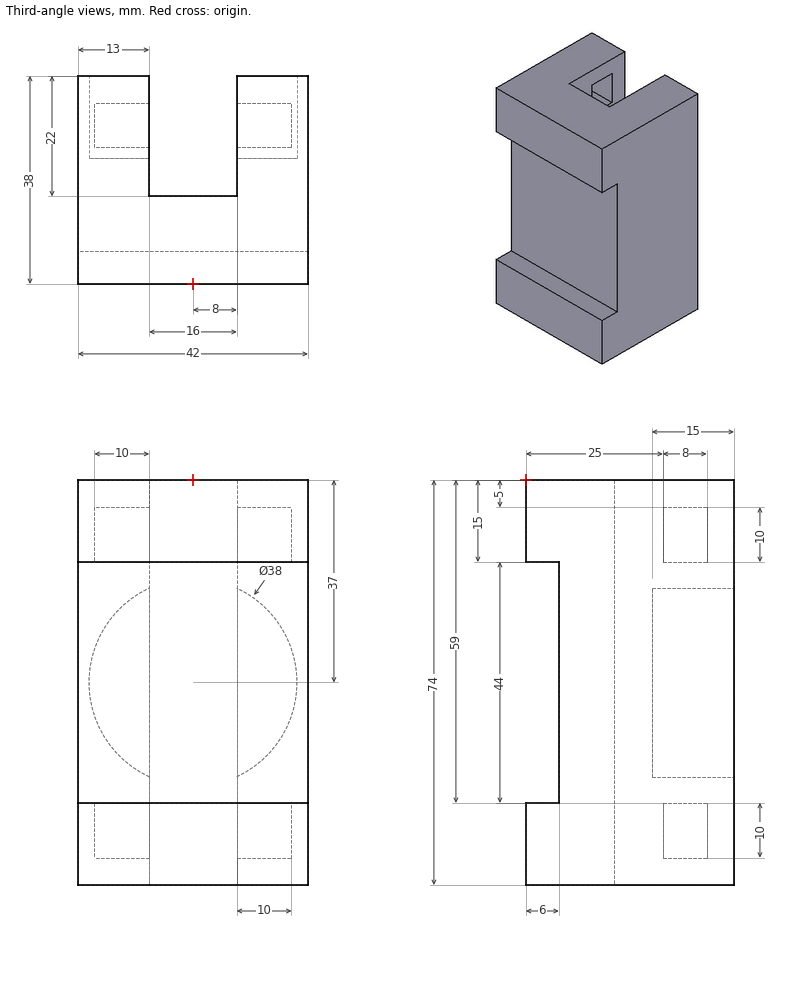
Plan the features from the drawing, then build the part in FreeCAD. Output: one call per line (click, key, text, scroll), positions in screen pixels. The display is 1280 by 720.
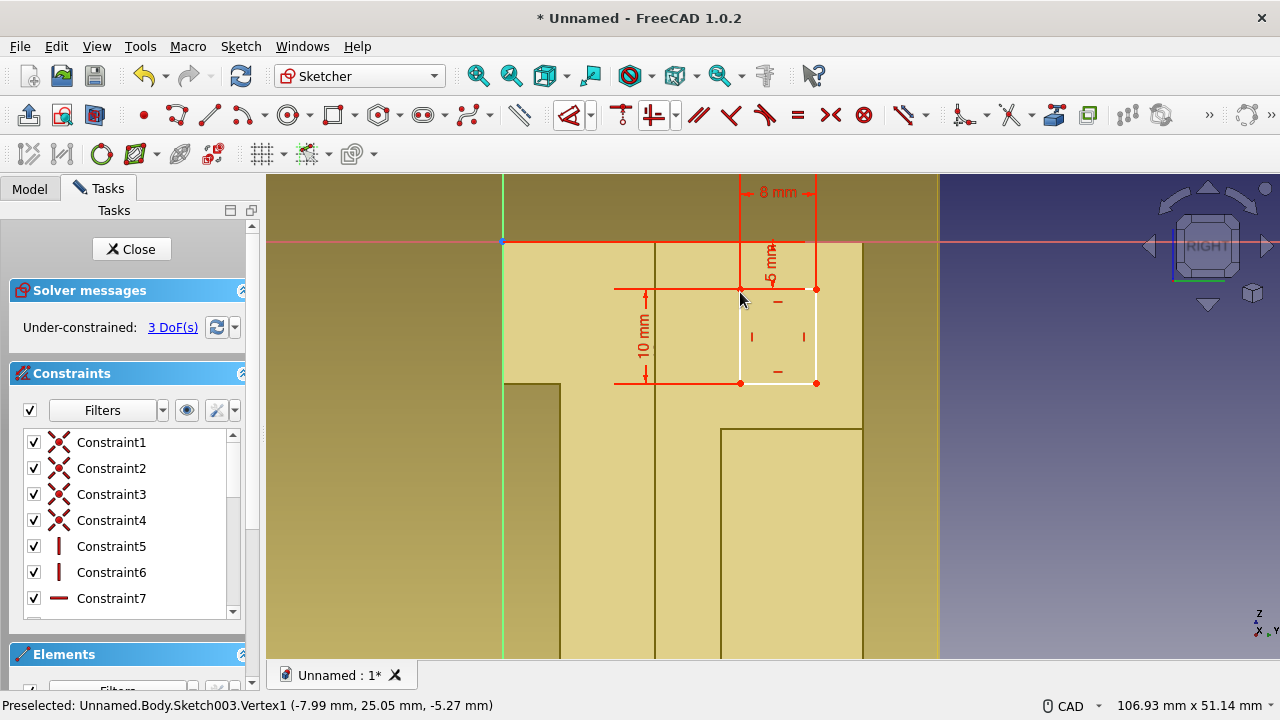
click(740, 289)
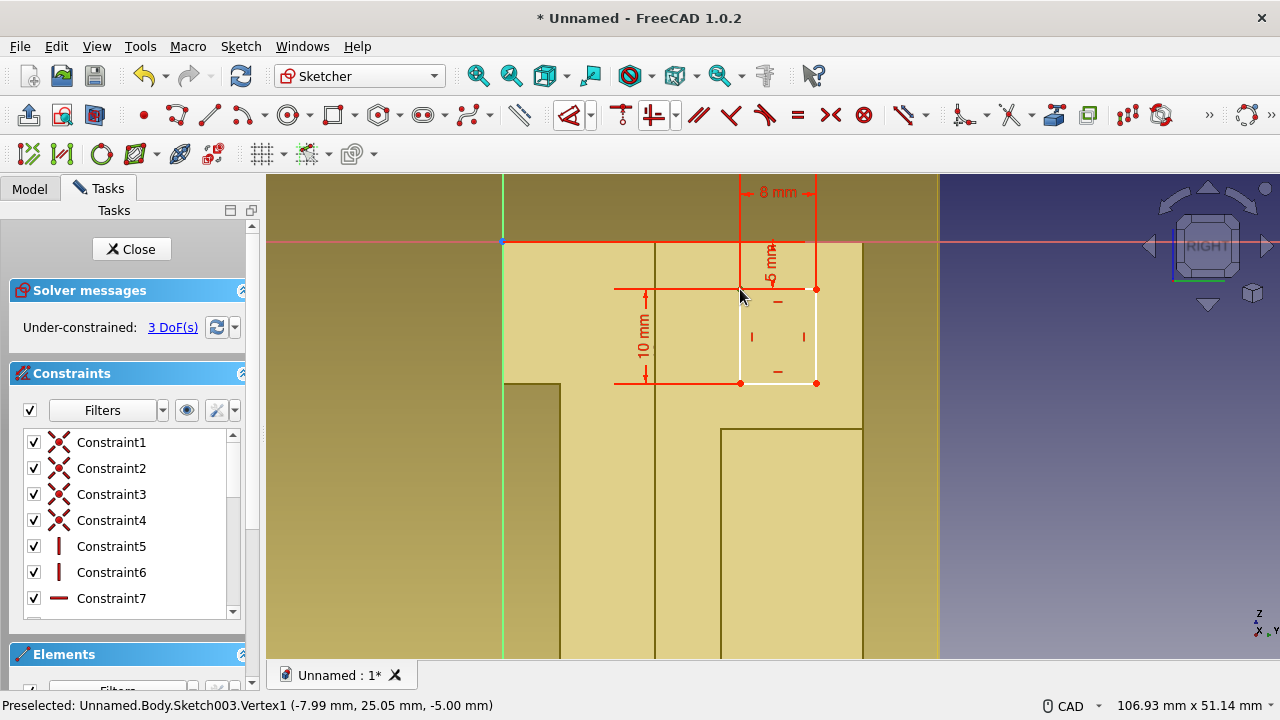
key(l)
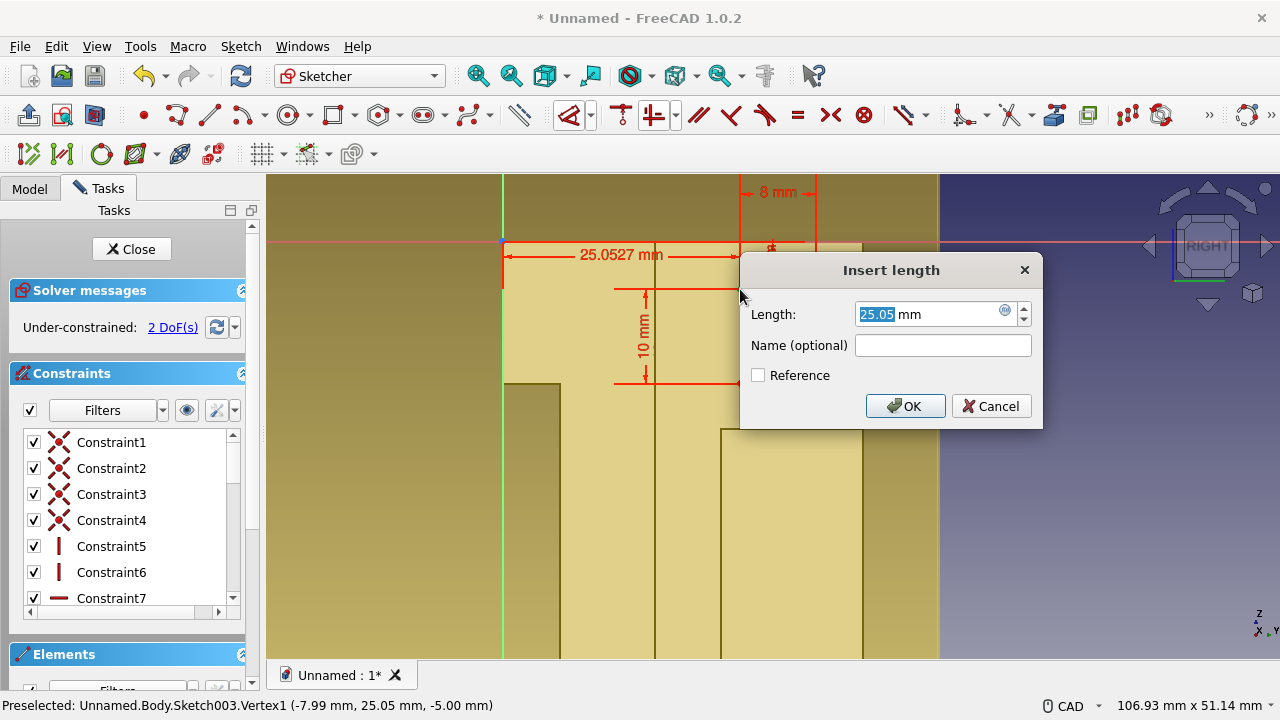
text(25)
key(Return)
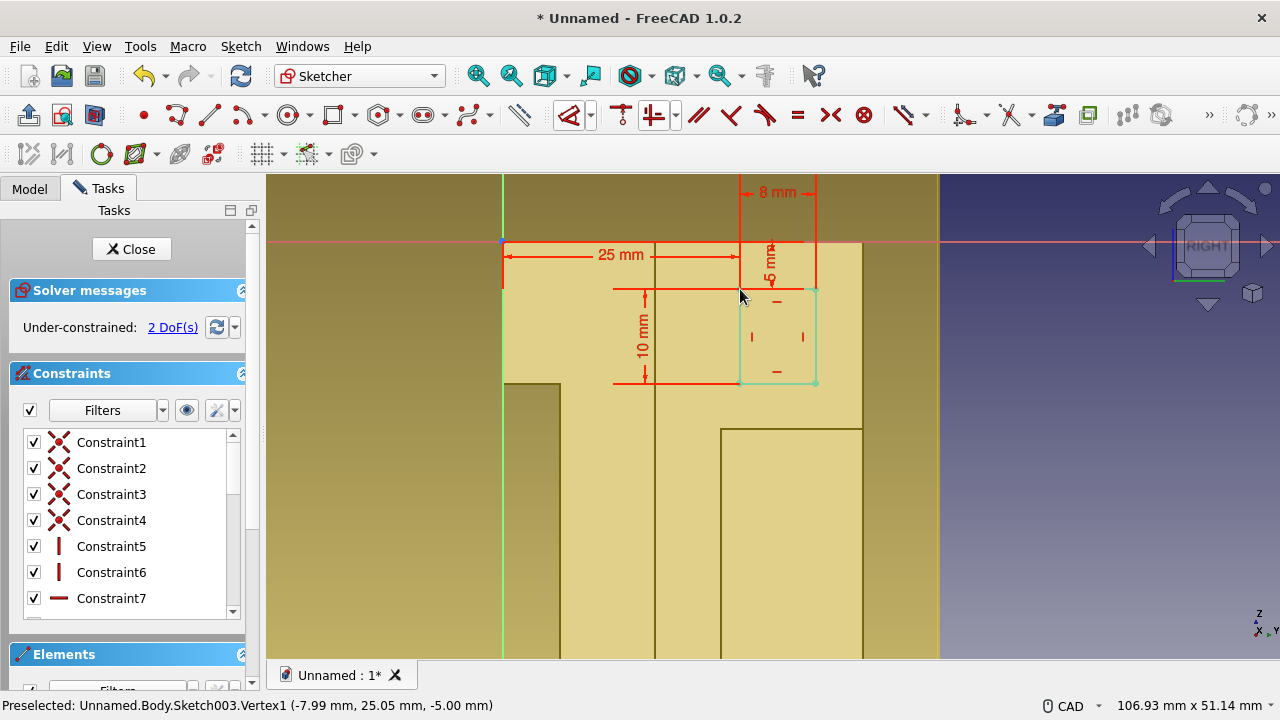
scroll(741, 292, down, 4)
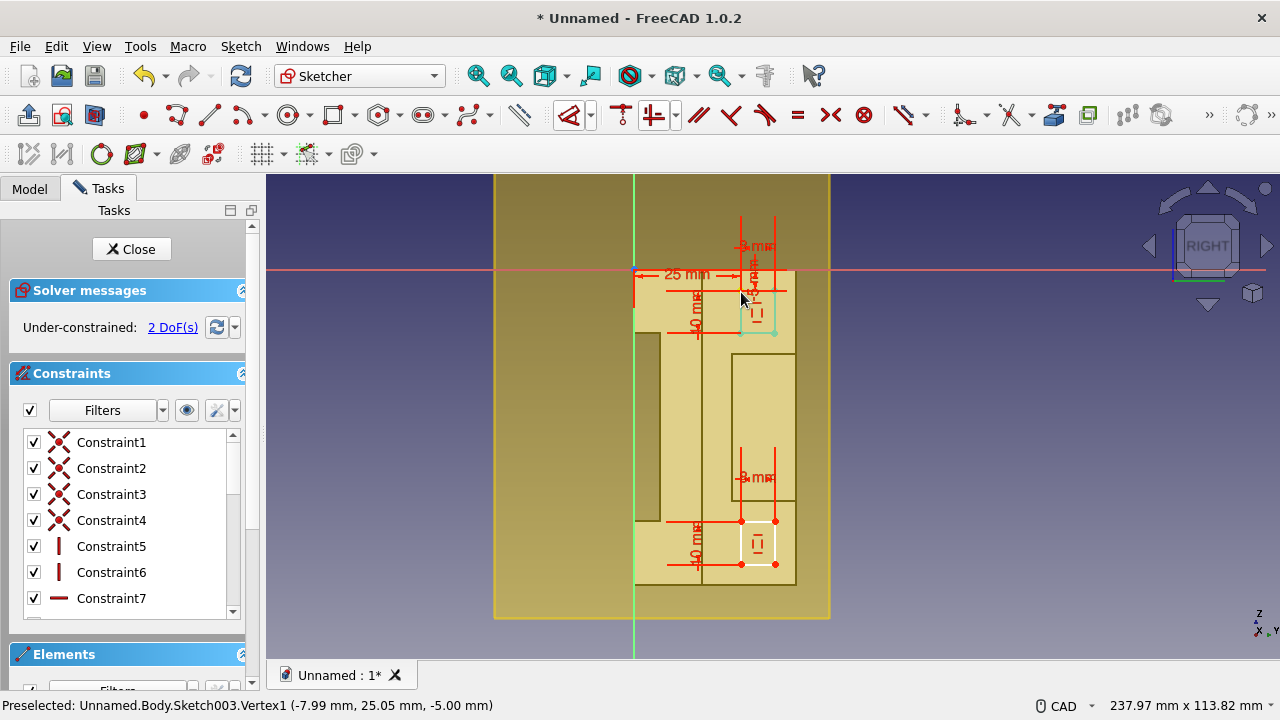
click(741, 522)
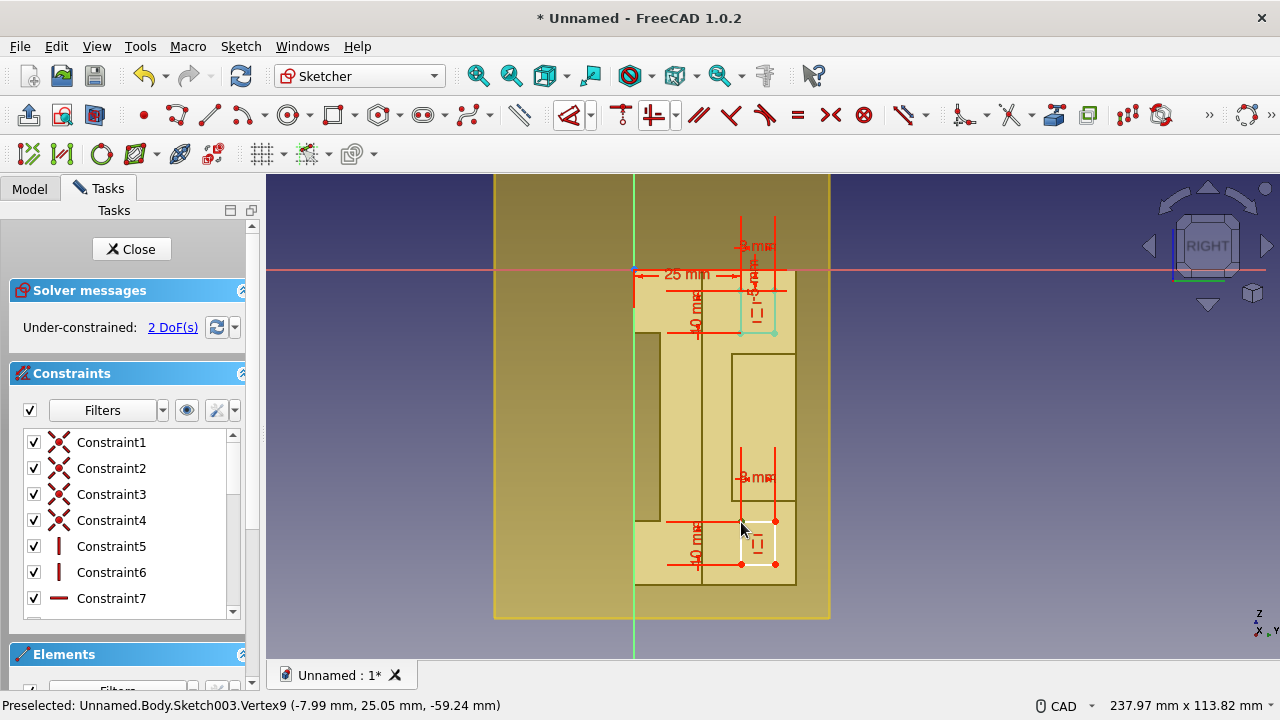
click(590, 116)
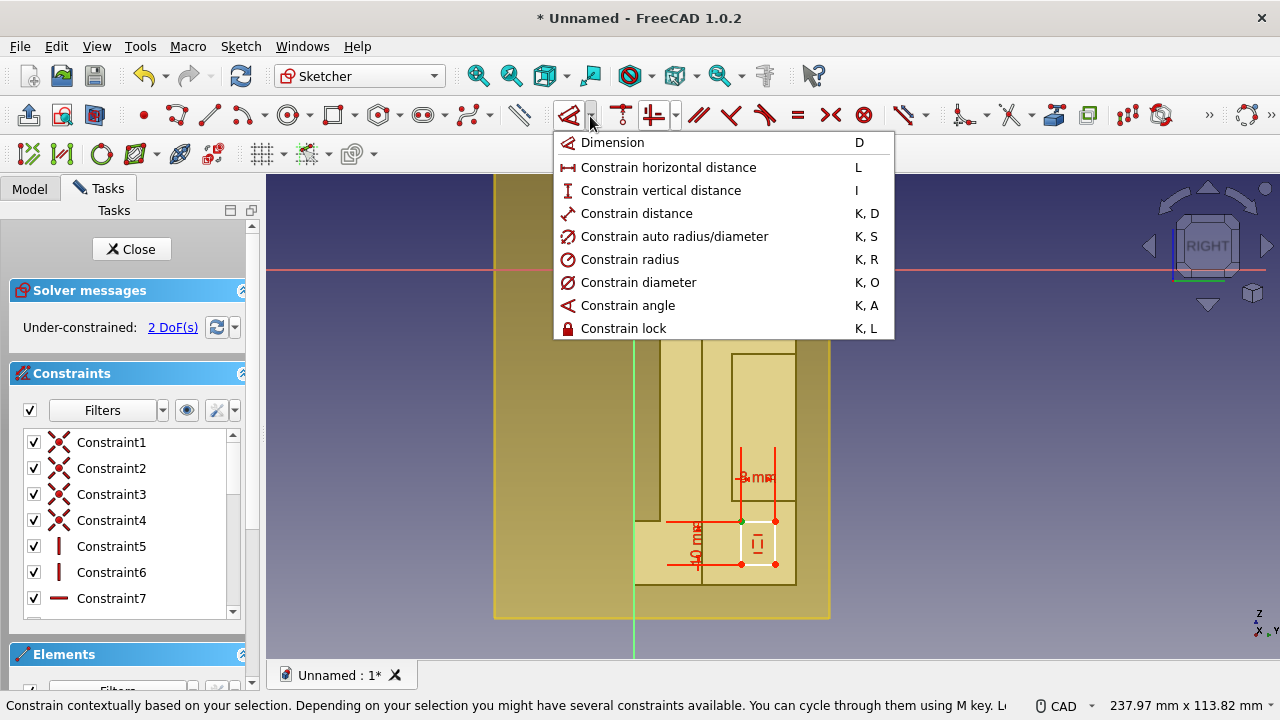
click(724, 168)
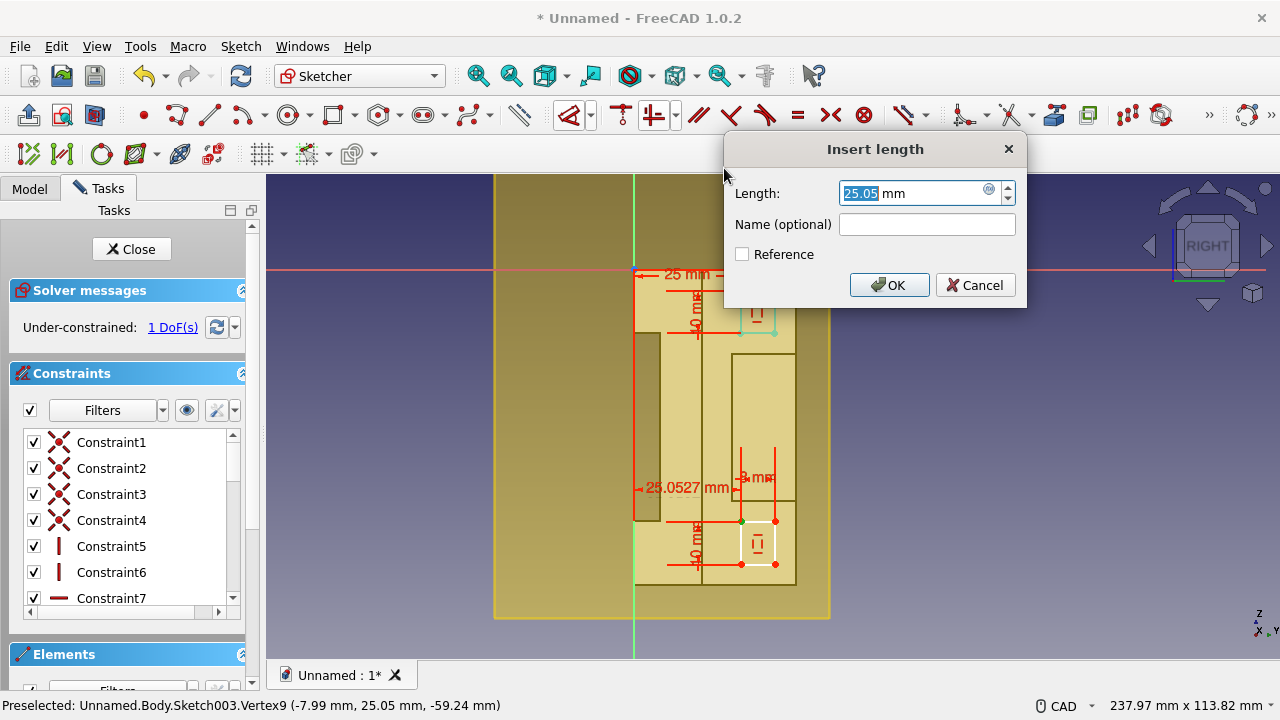
text(25)
key(Return)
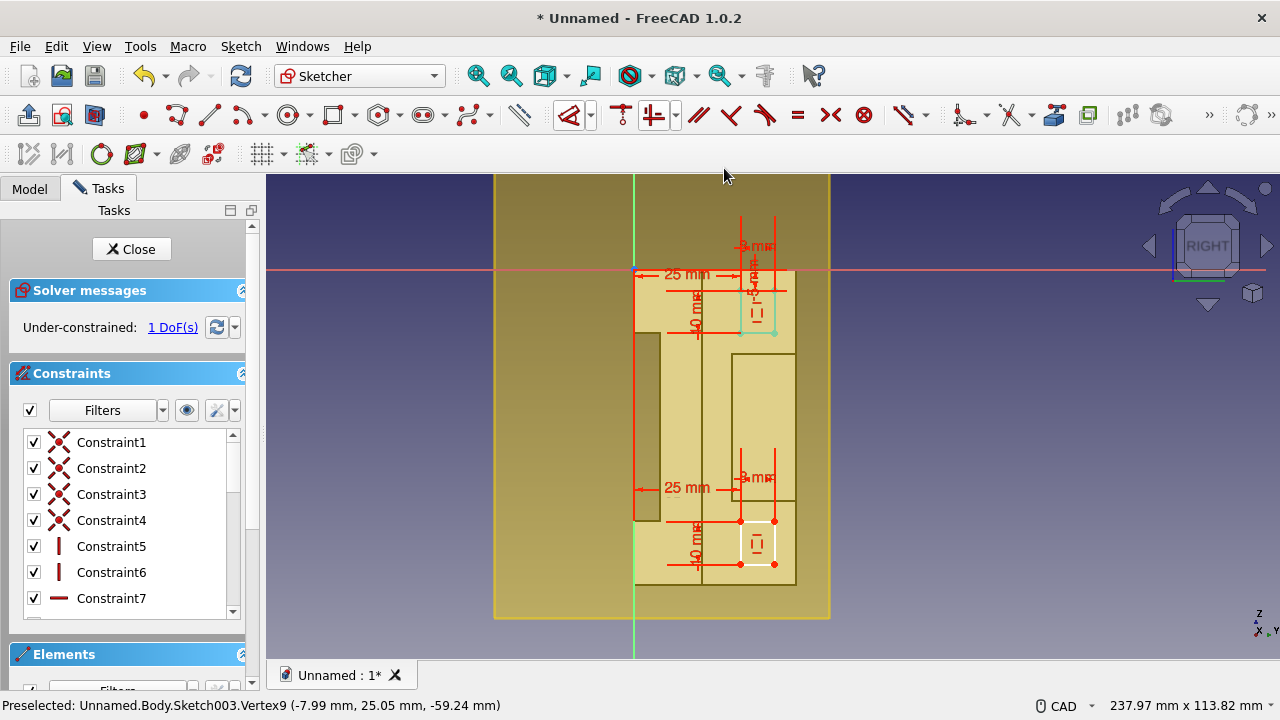
click(741, 522)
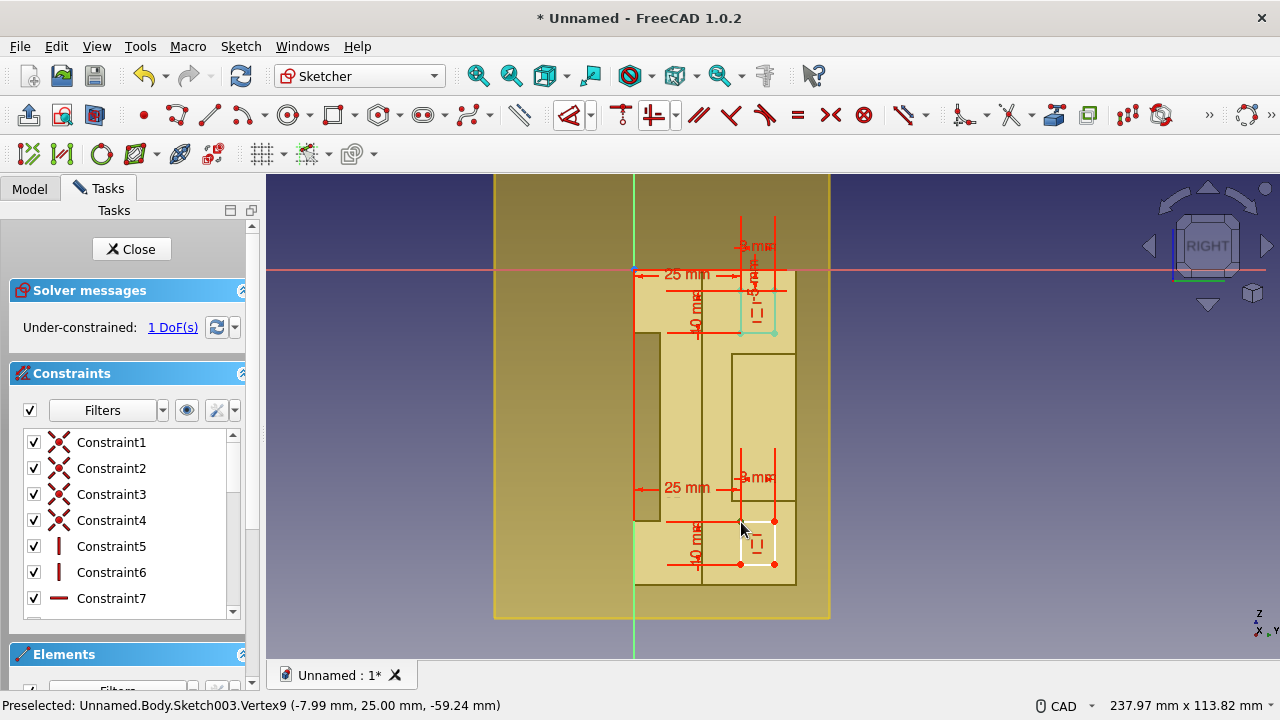
key(i)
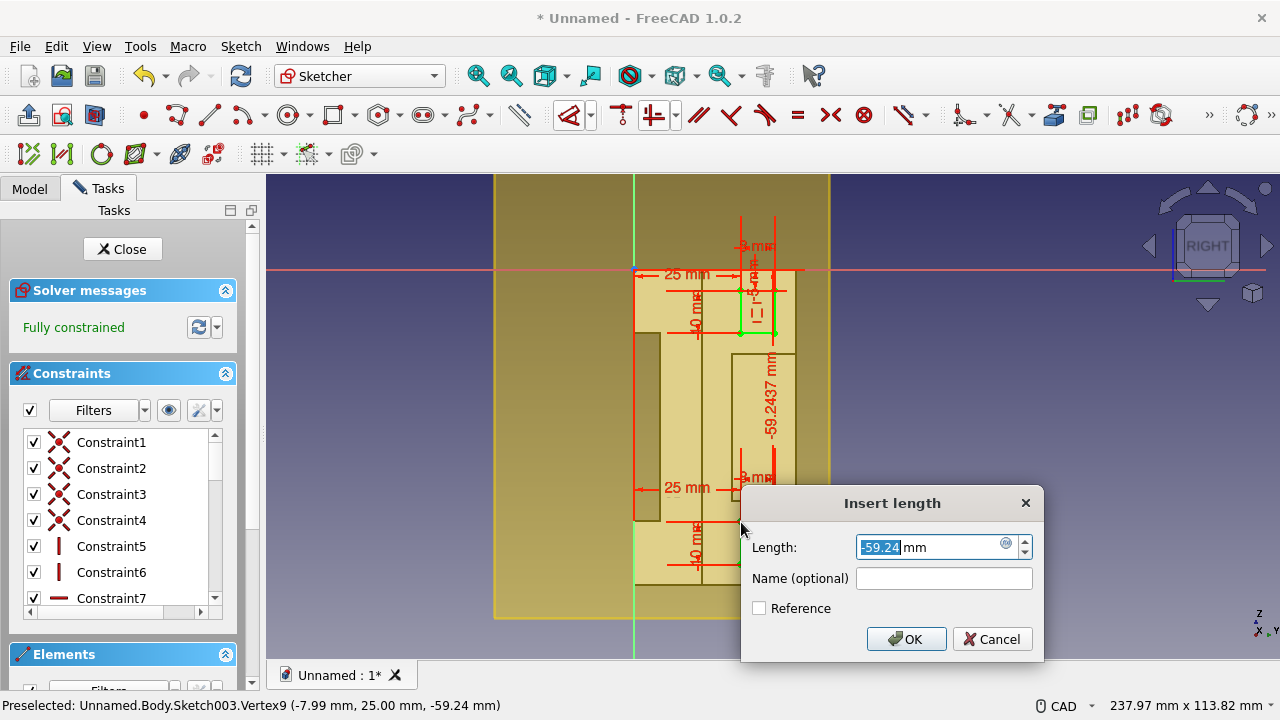
text(-59)
key(Return)